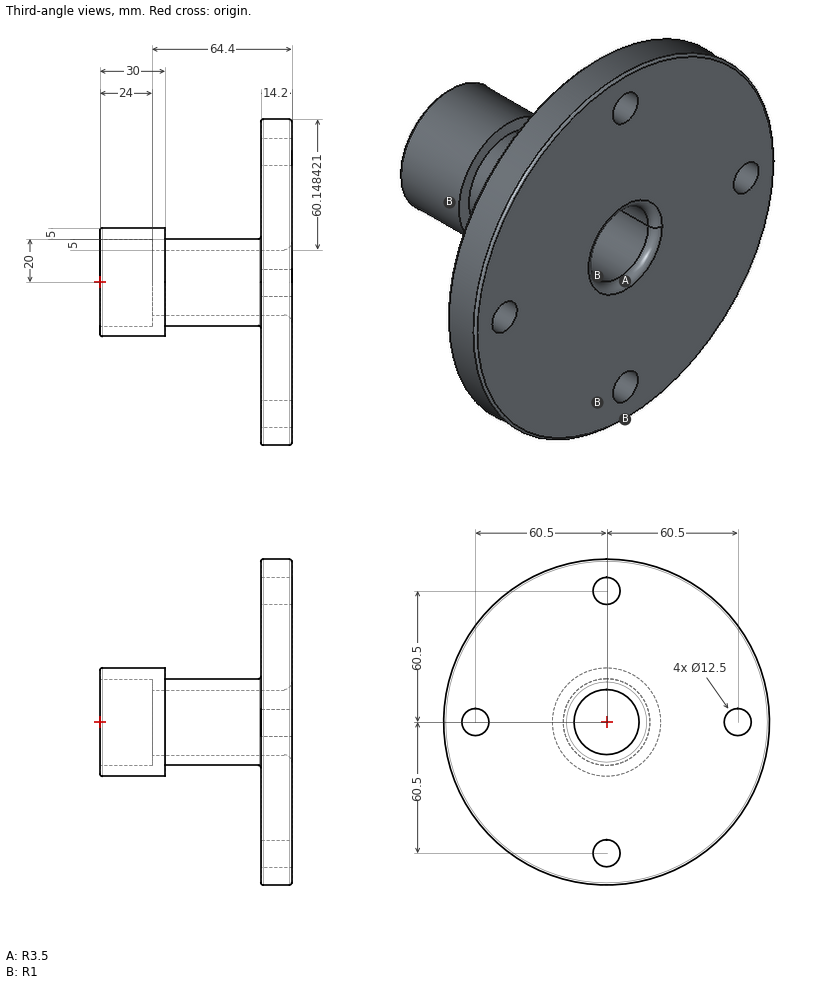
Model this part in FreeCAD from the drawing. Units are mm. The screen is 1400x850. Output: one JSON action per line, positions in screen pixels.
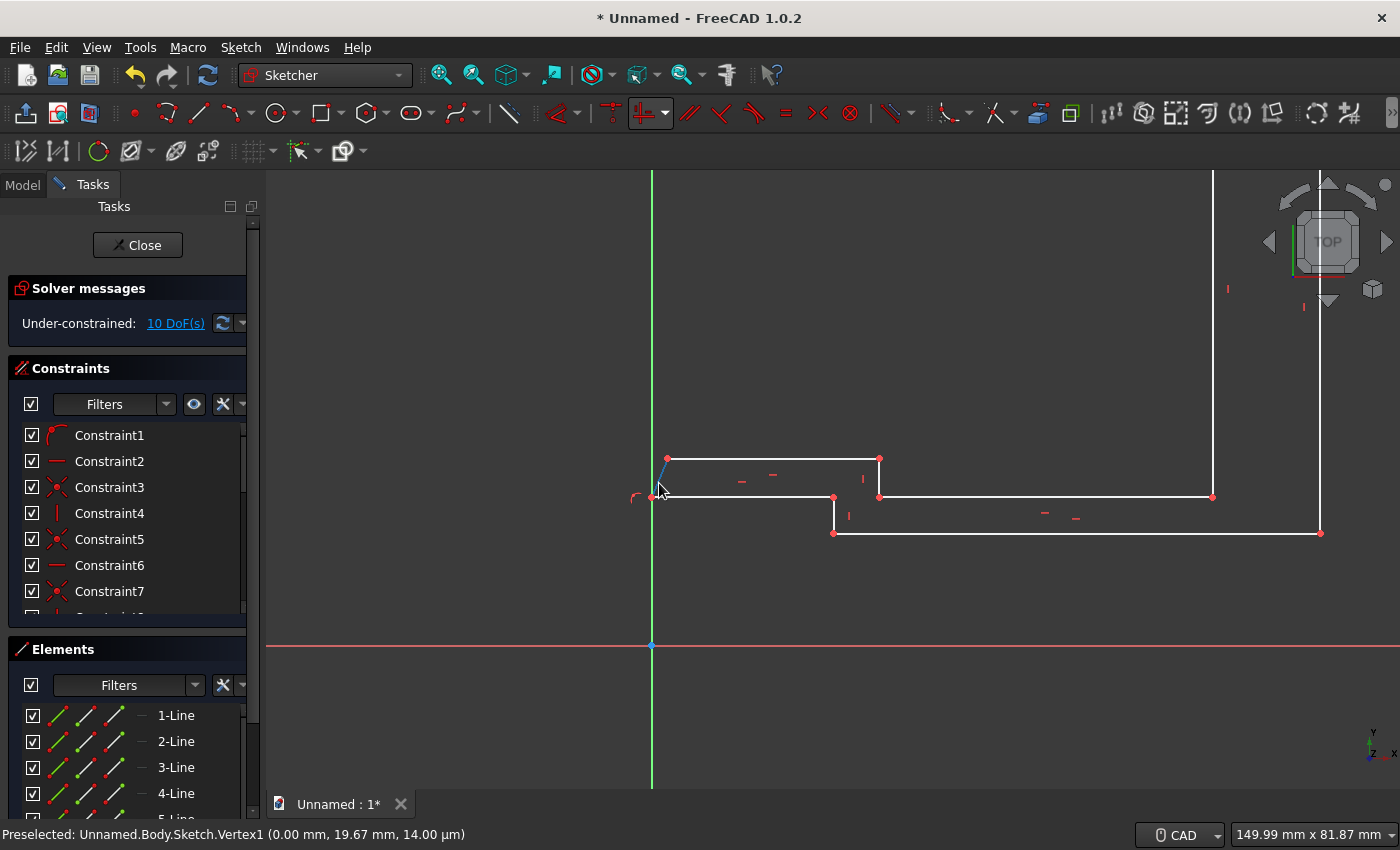
{"action": "left_click", "coordinate": [658, 482]}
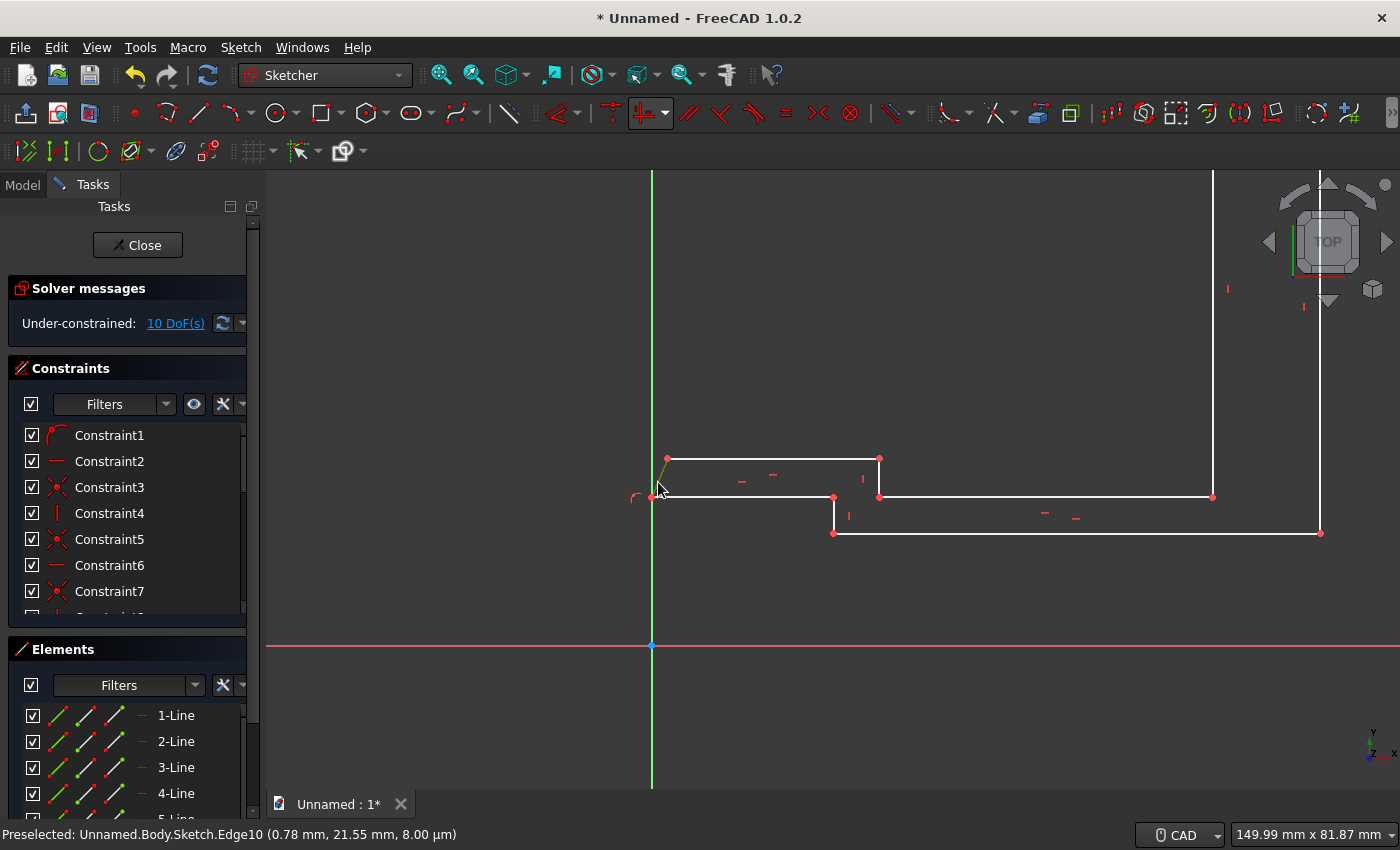
{"action": "key", "text": "v"}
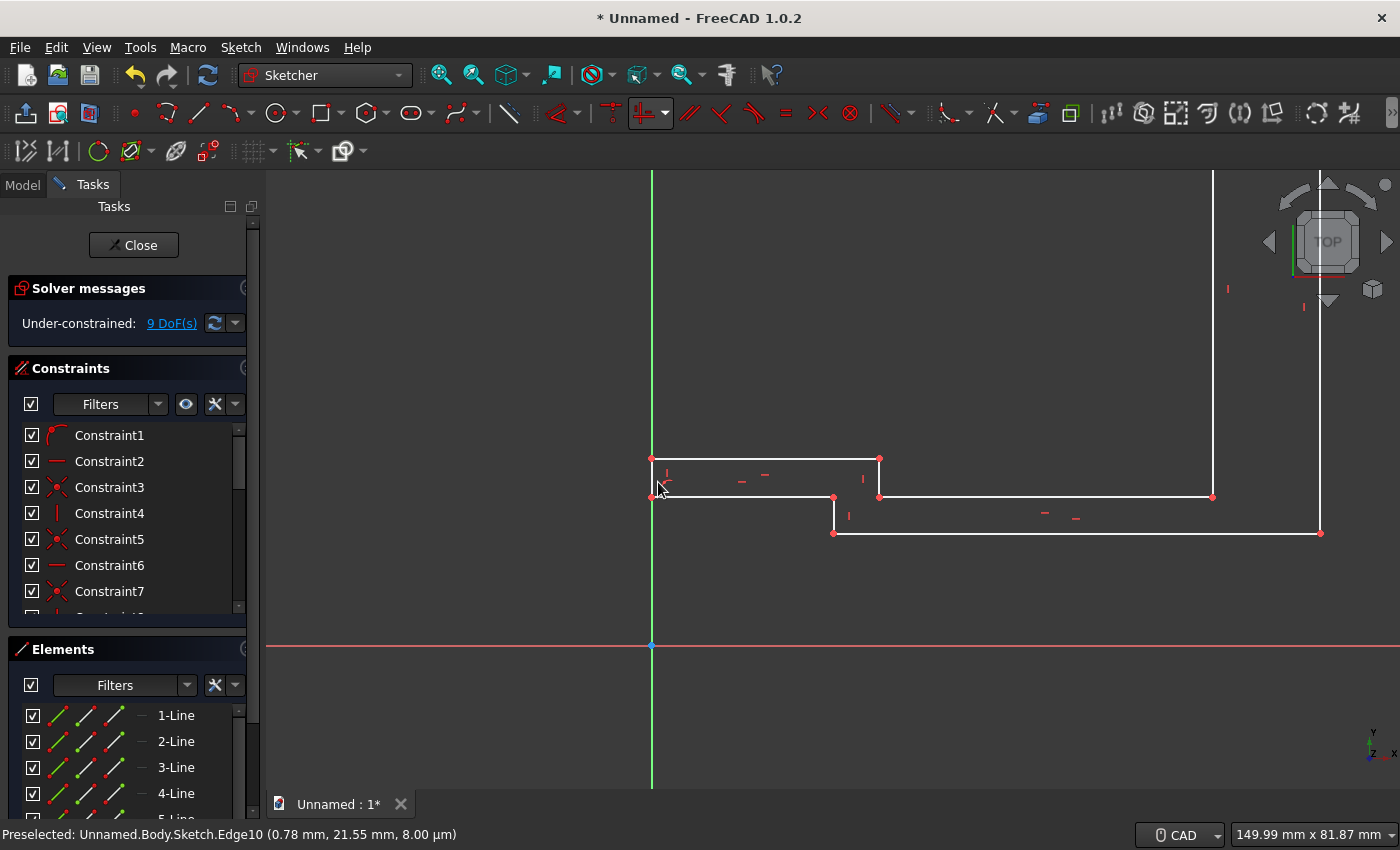
{"action": "left_click", "coordinate": [556, 114]}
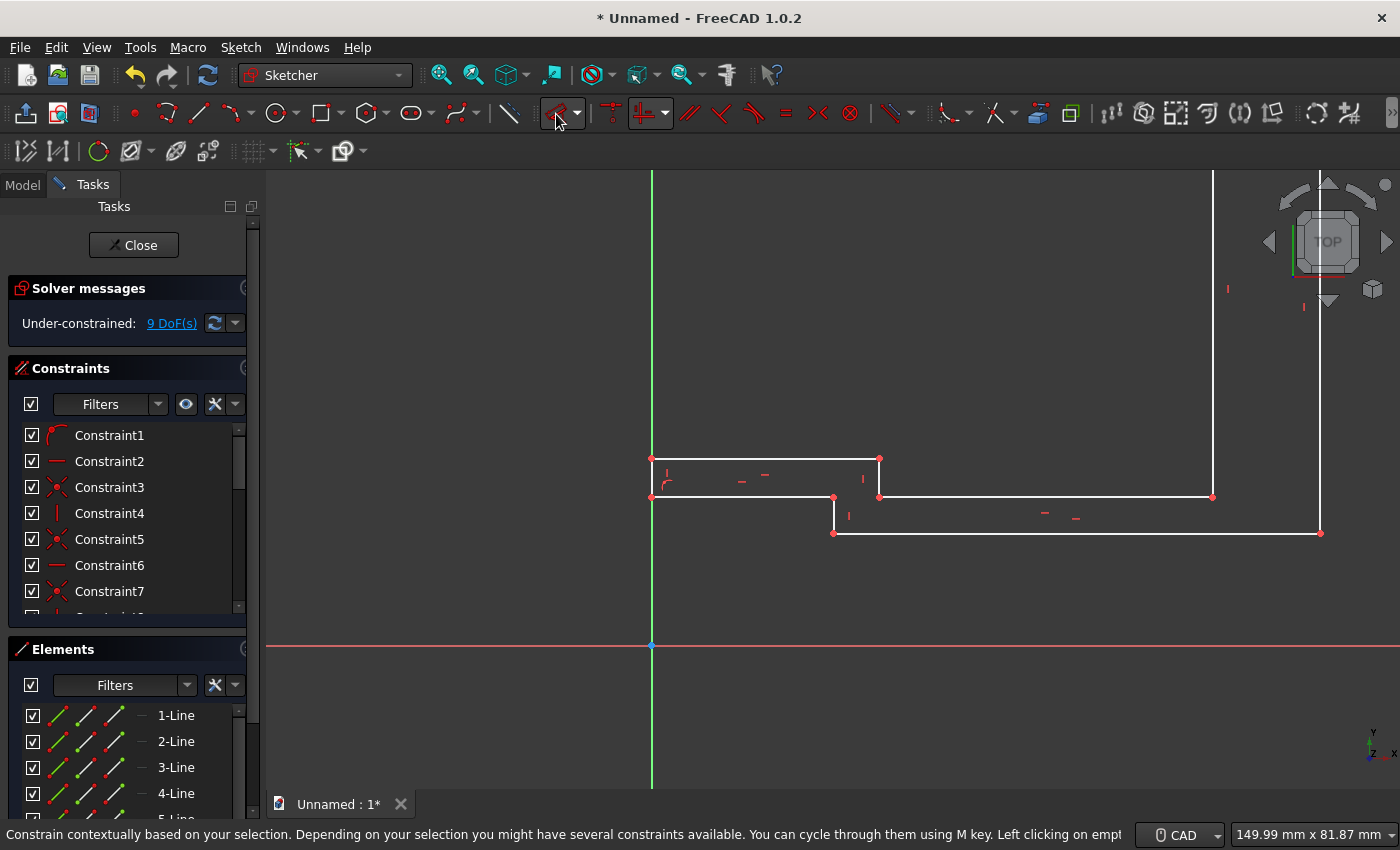
{"action": "scroll", "coordinate": [834, 508], "scroll_direction": "up", "scroll_amount": 2}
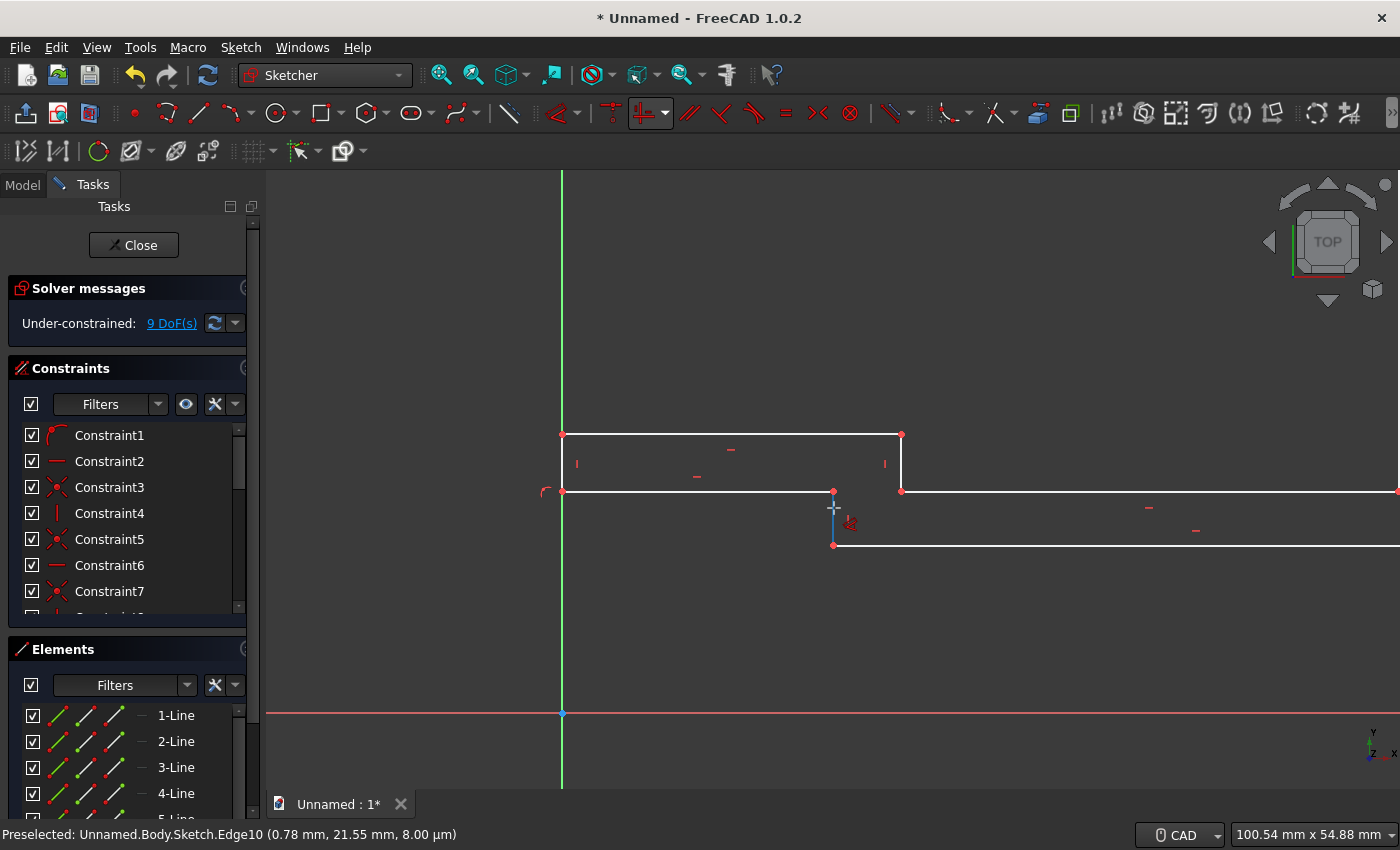
{"action": "left_click", "coordinate": [833, 508]}
{"action": "left_click", "coordinate": [799, 519]}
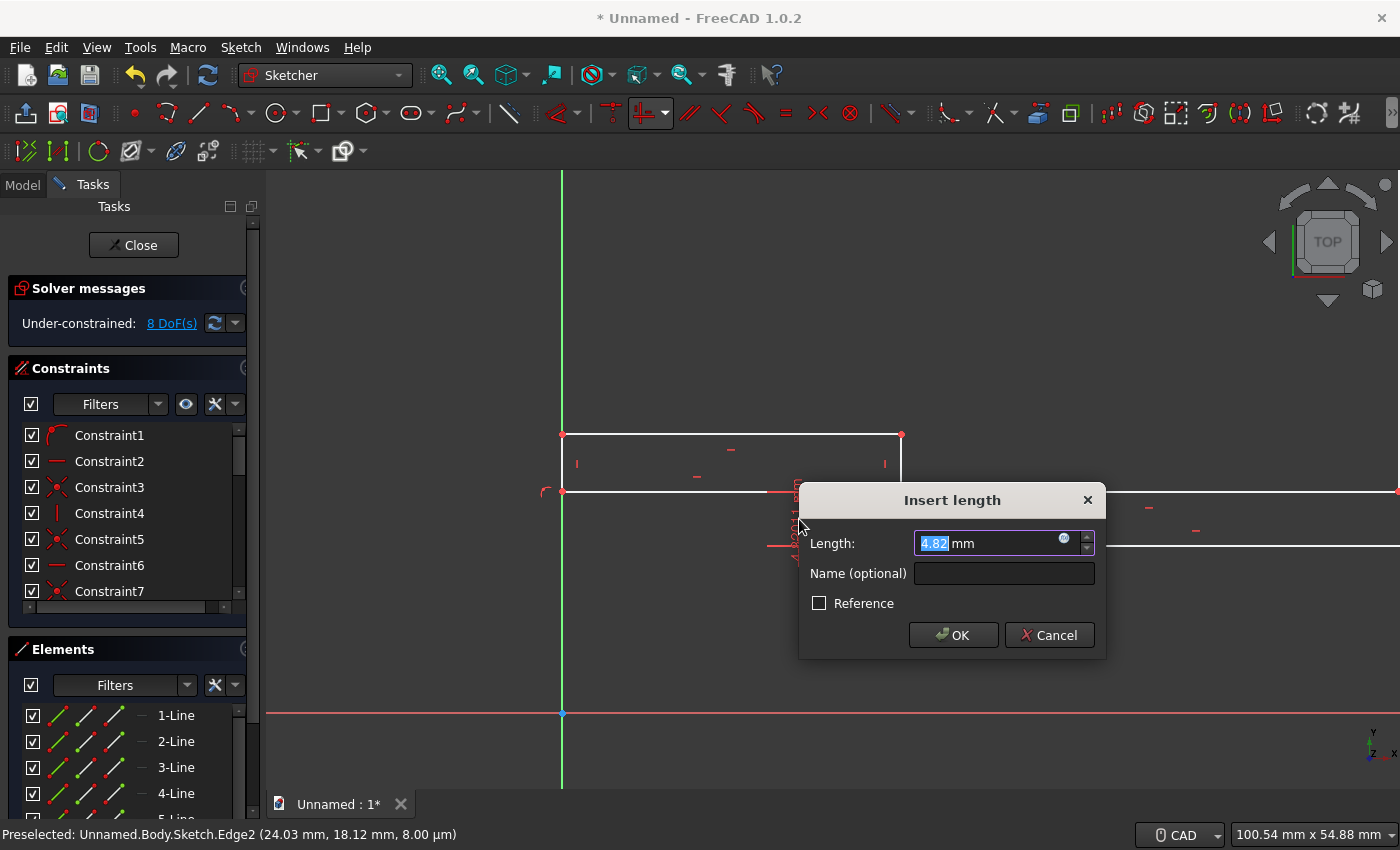
{"action": "type", "text": "5"}
{"action": "key", "text": "Return"}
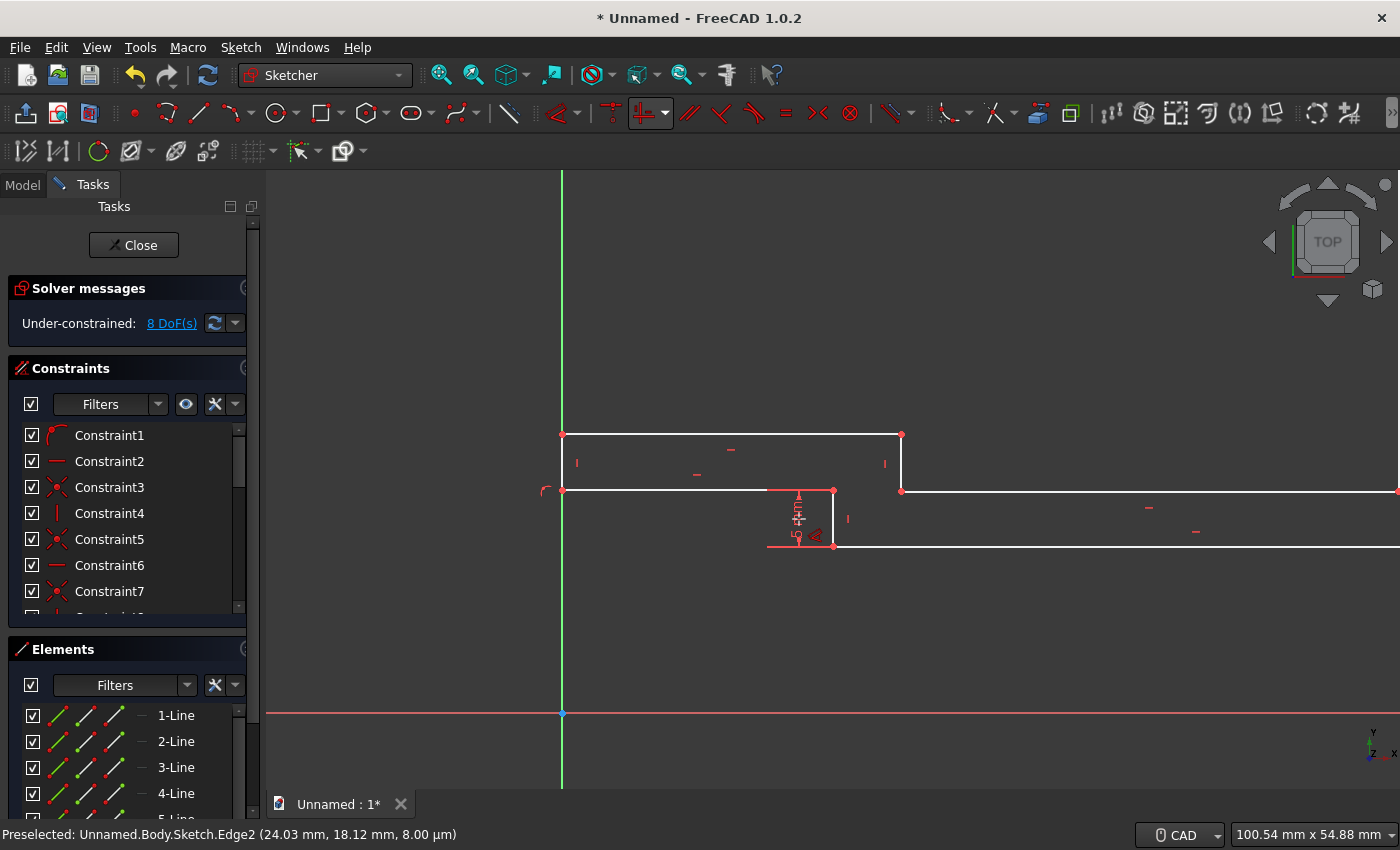
{"action": "left_click", "coordinate": [901, 474]}
{"action": "left_click", "coordinate": [867, 463]}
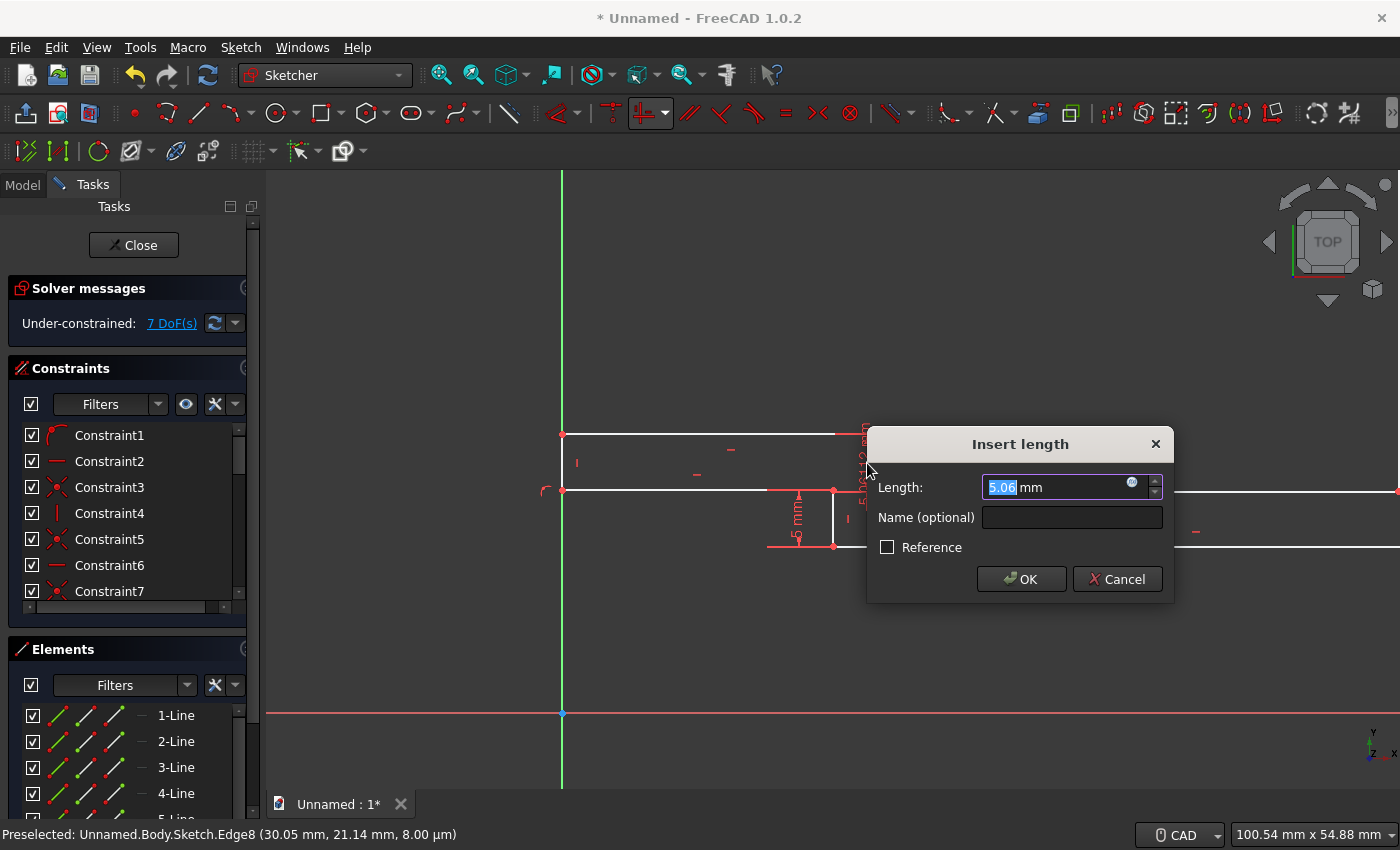
{"action": "type", "text": "5"}
{"action": "key", "text": "Return"}